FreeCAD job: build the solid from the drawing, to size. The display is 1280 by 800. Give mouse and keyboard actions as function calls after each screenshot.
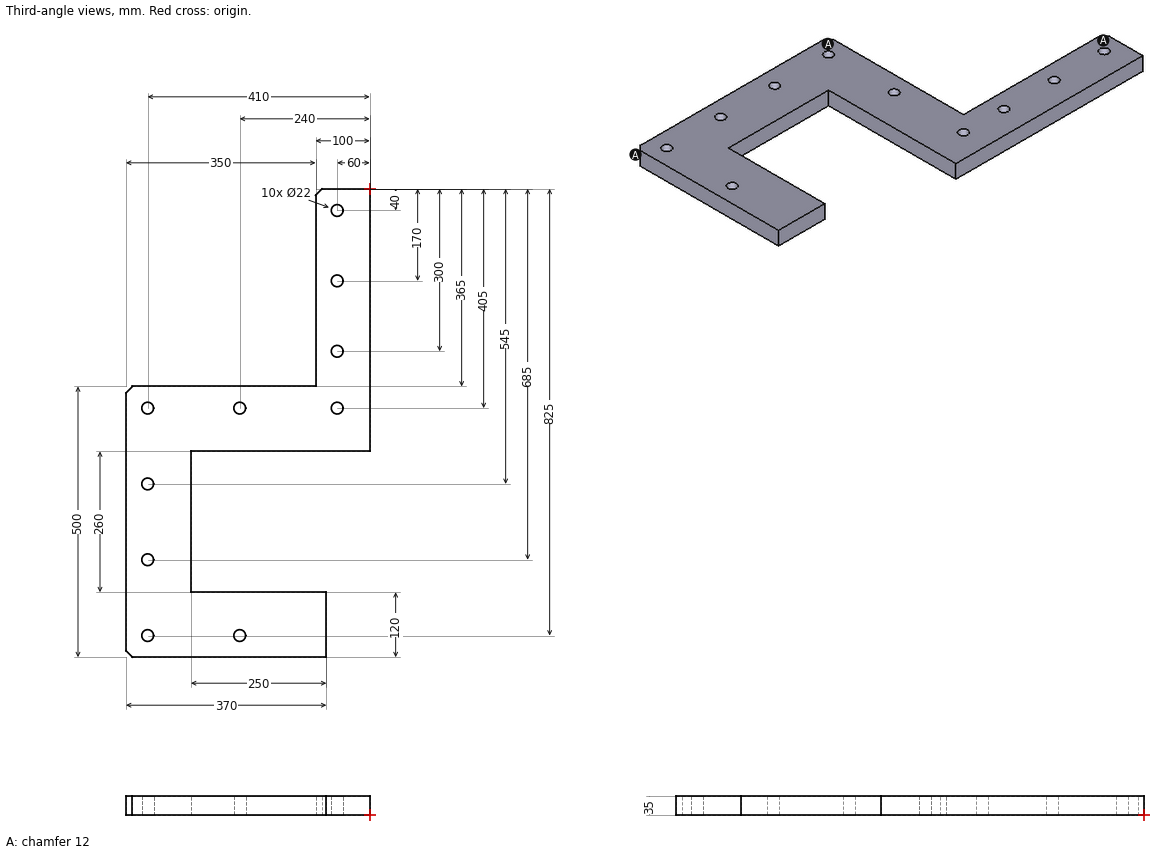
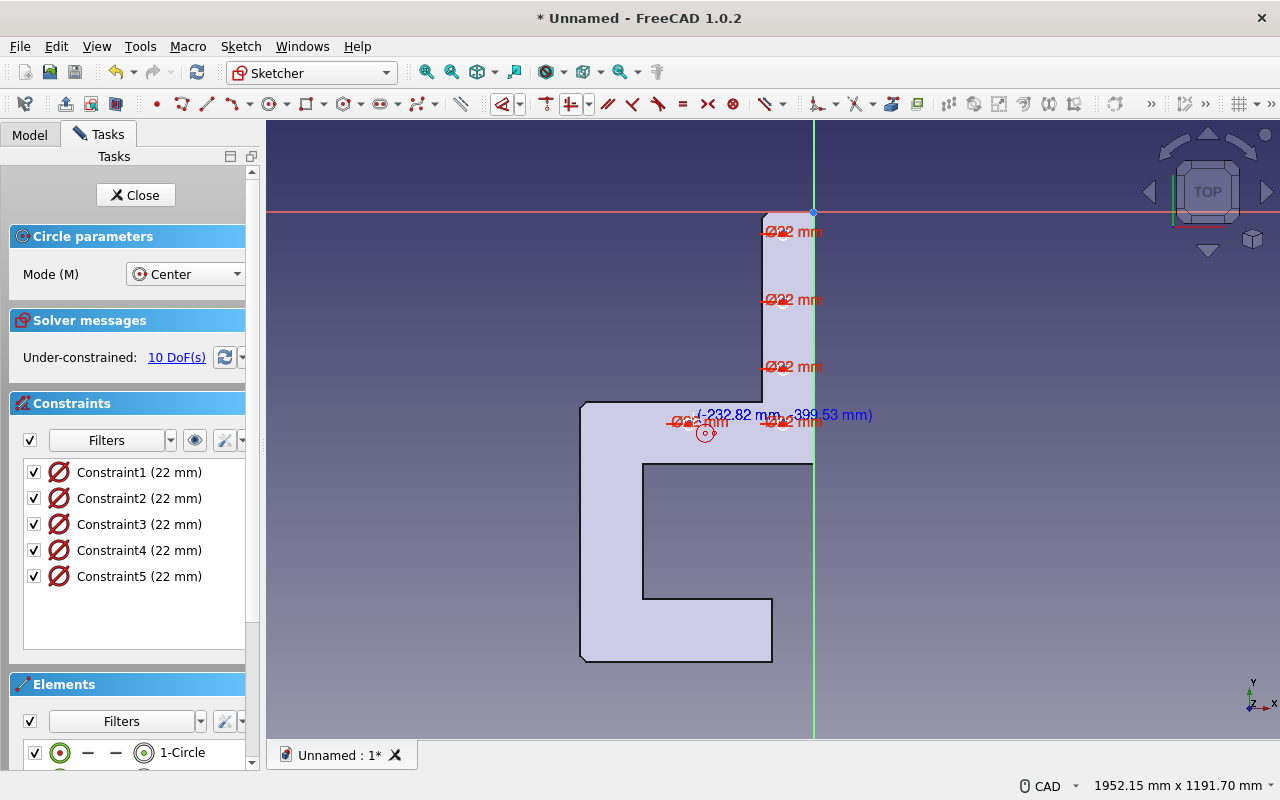
scroll(601, 423, up, 7)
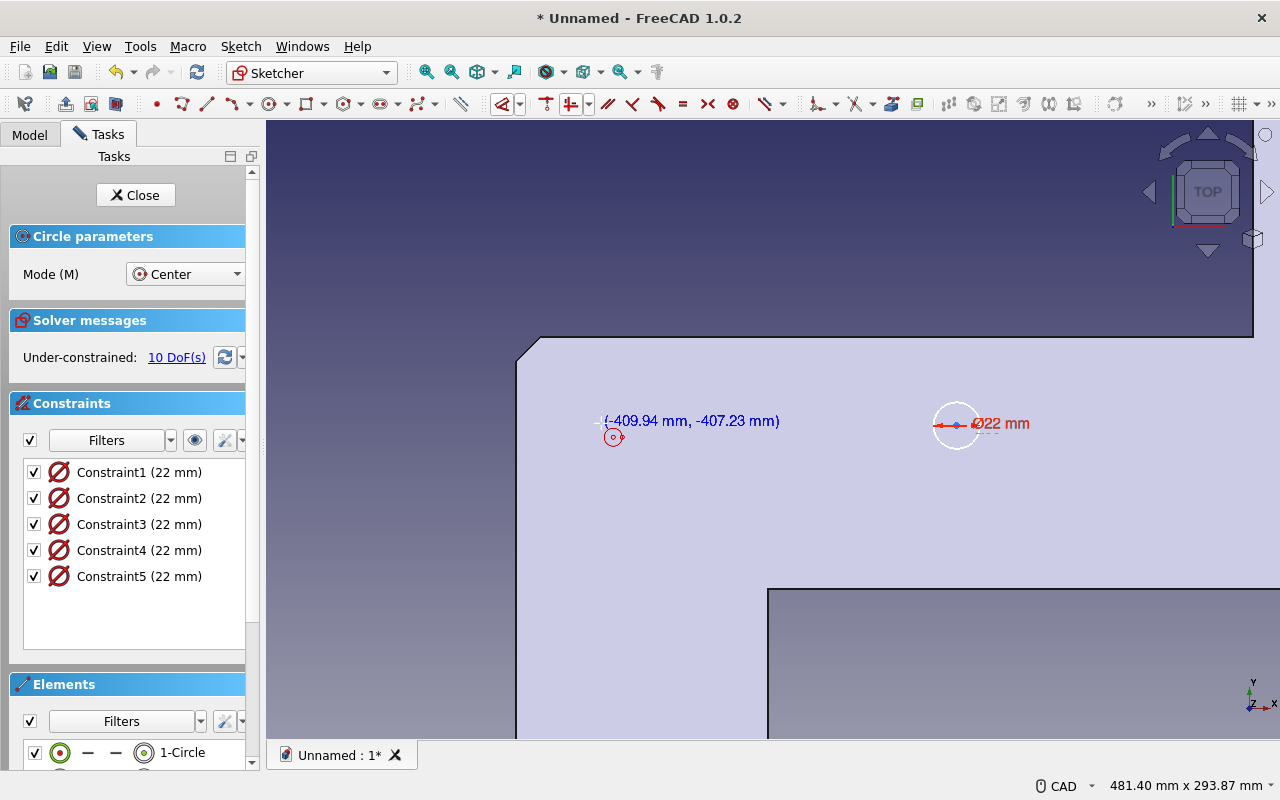
scroll(601, 423, down, 7)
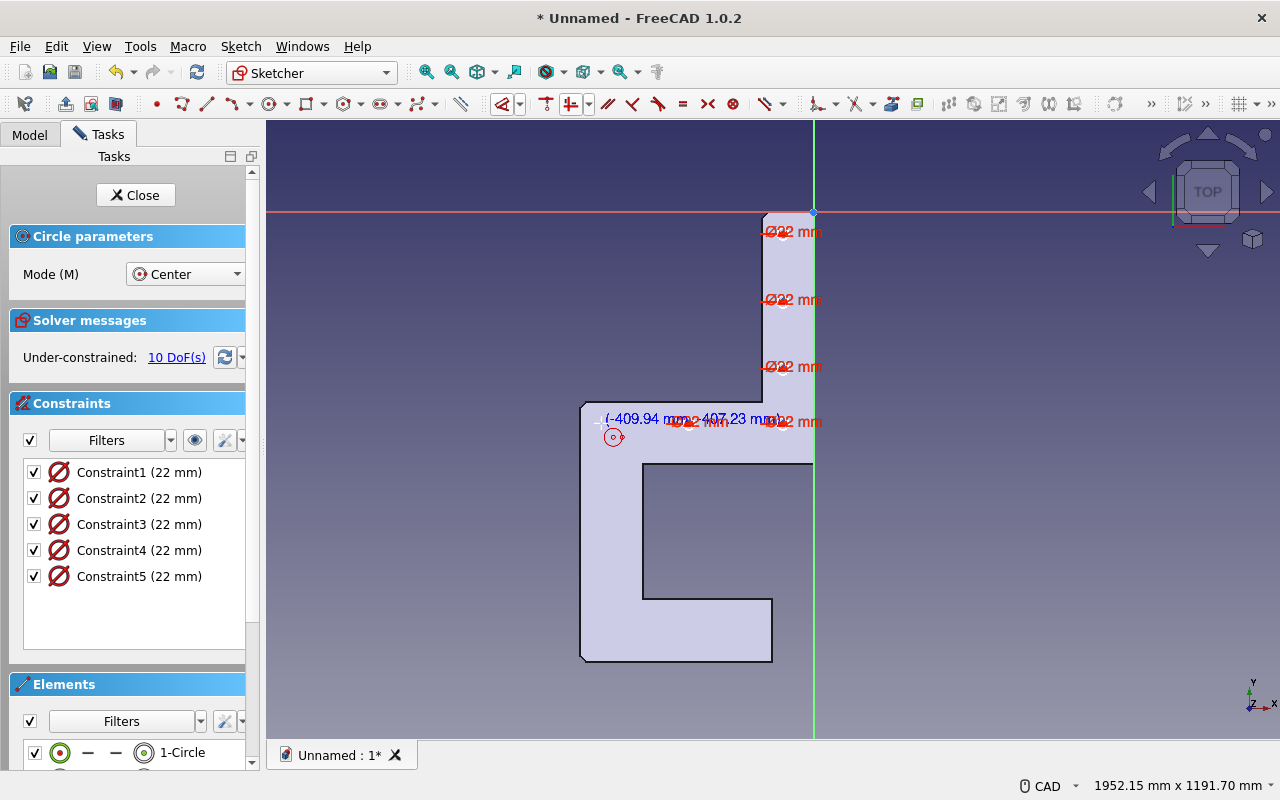
click(601, 423)
move(605, 419)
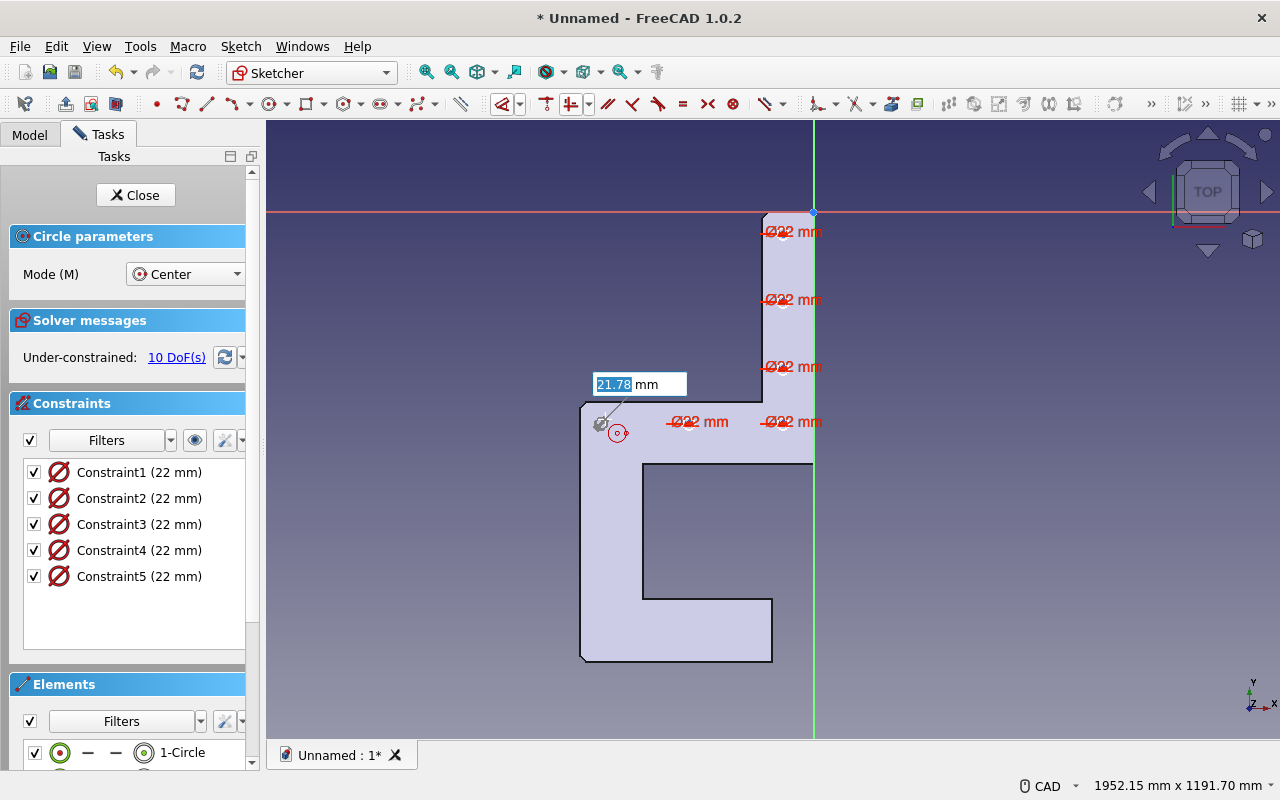
text(22)
key(Return)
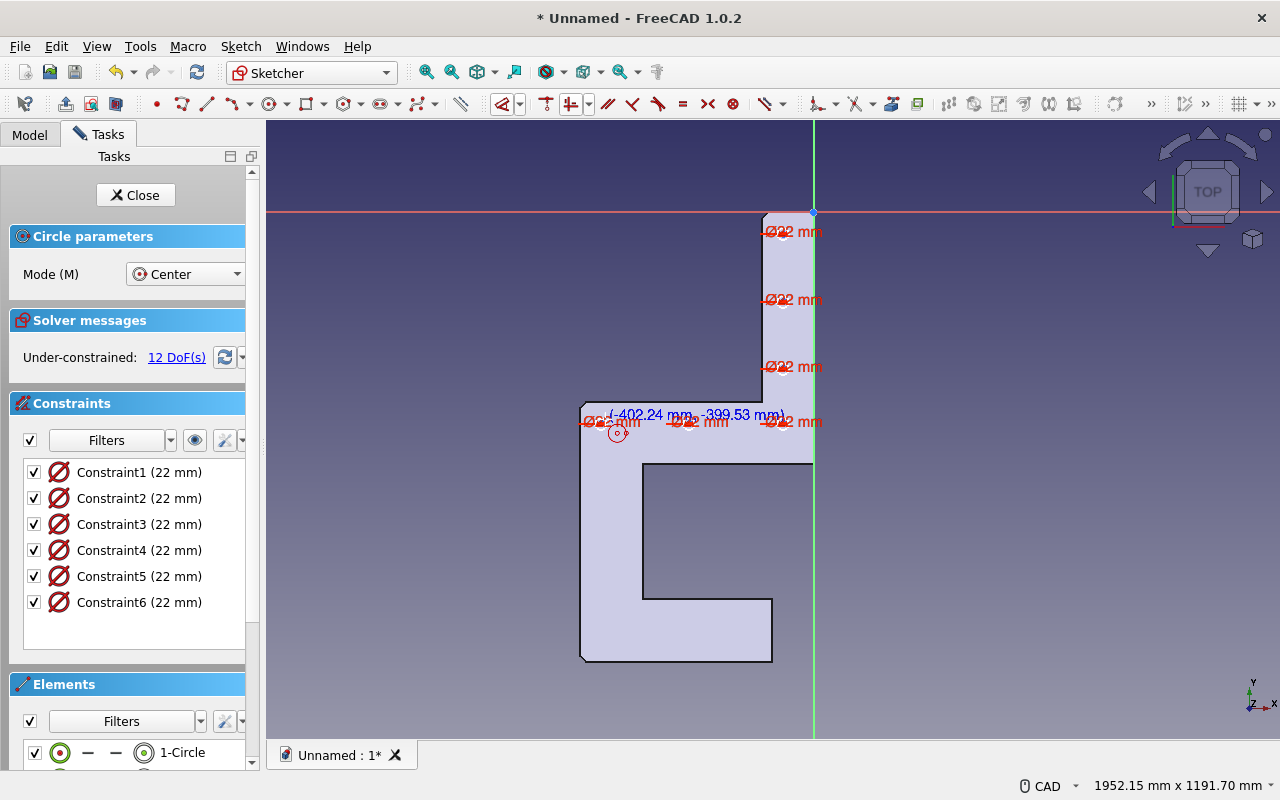
scroll(601, 496, up, 7)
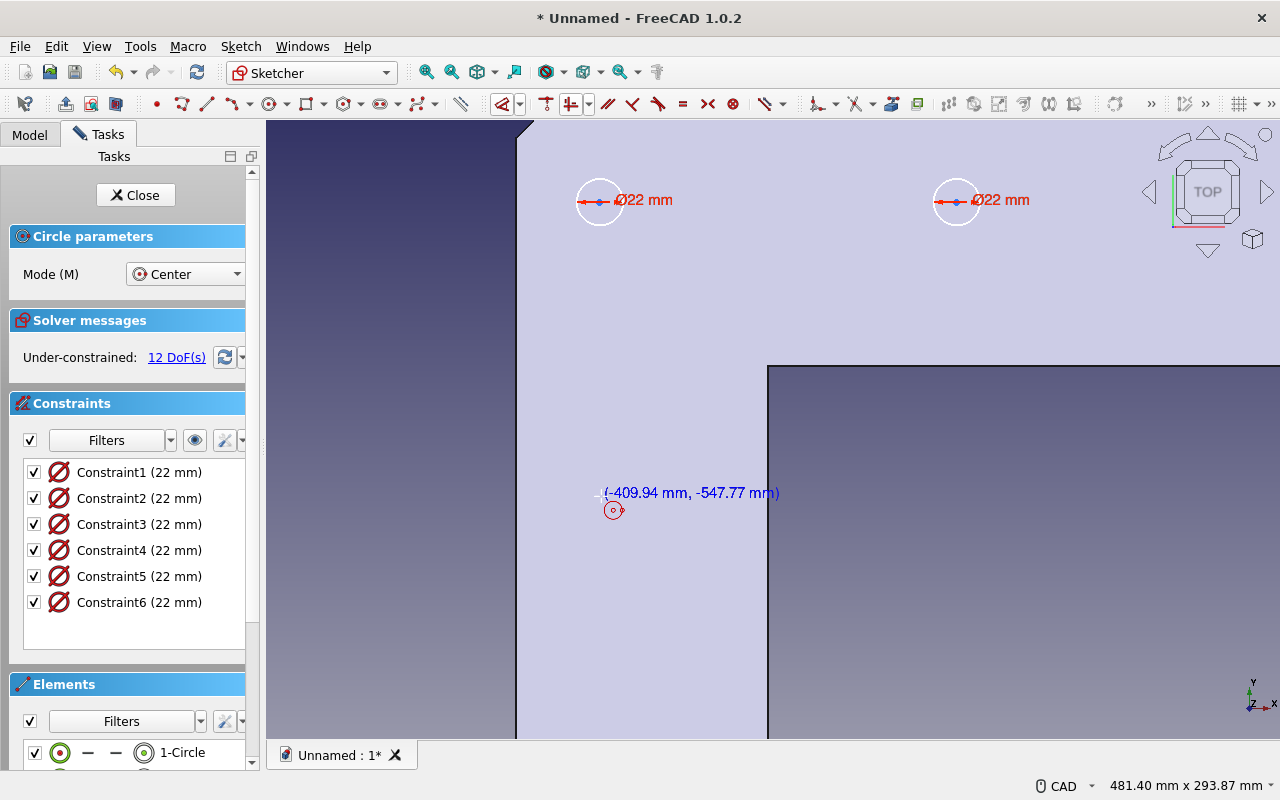
scroll(601, 496, down, 7)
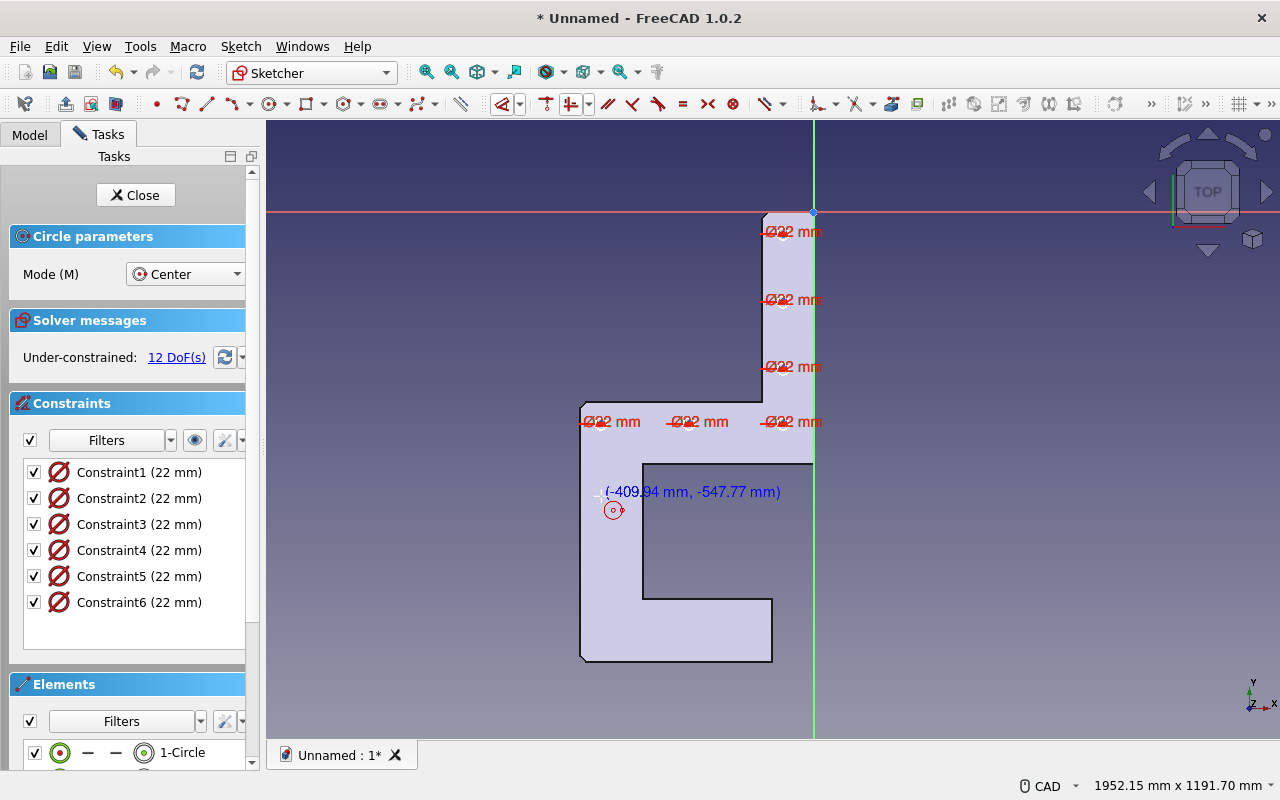
click(601, 496)
move(605, 492)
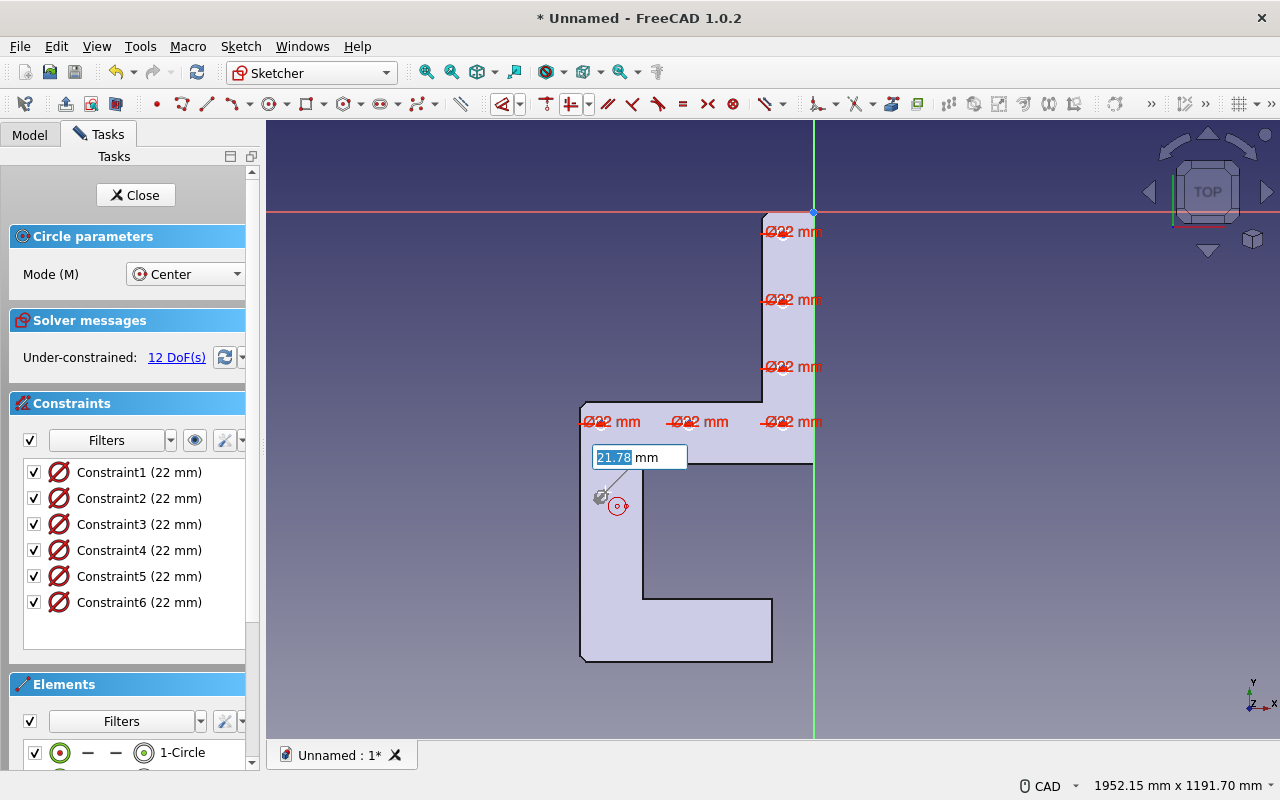
text(22)
key(Return)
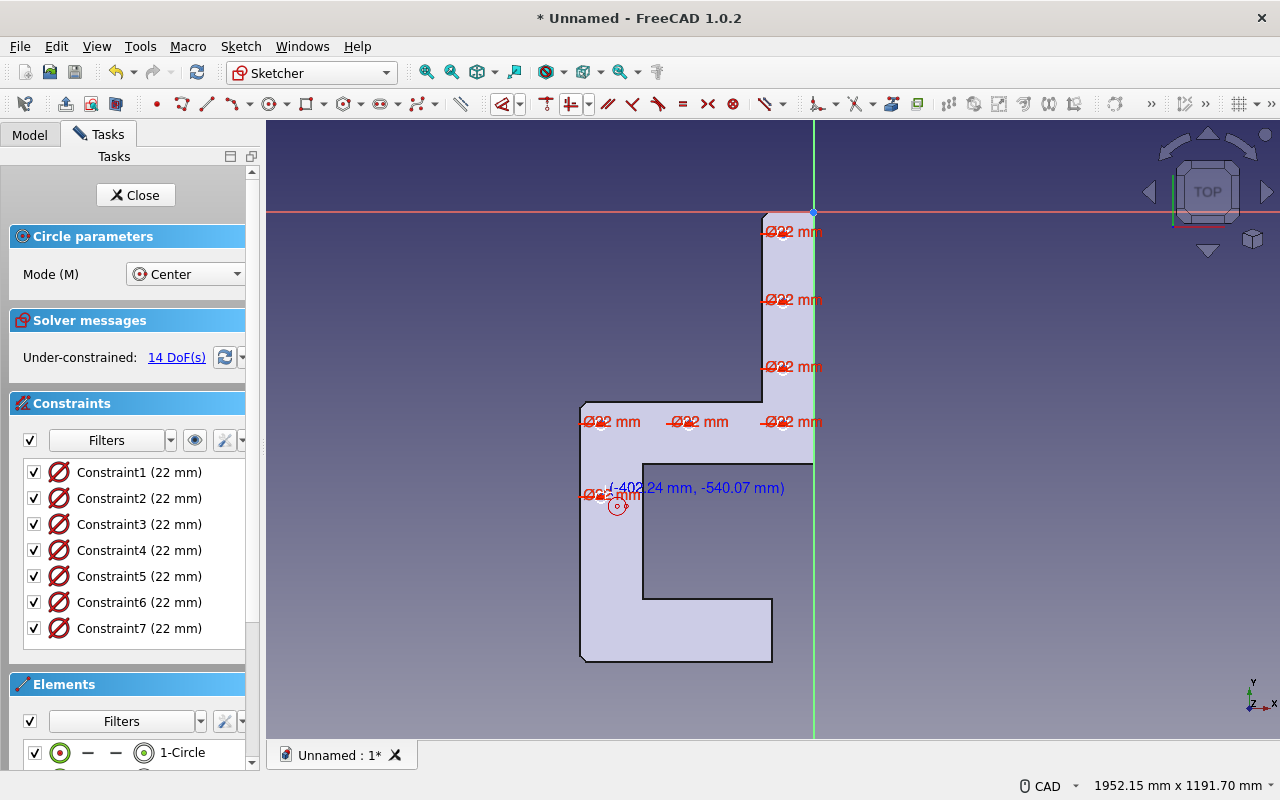
scroll(601, 568, up, 7)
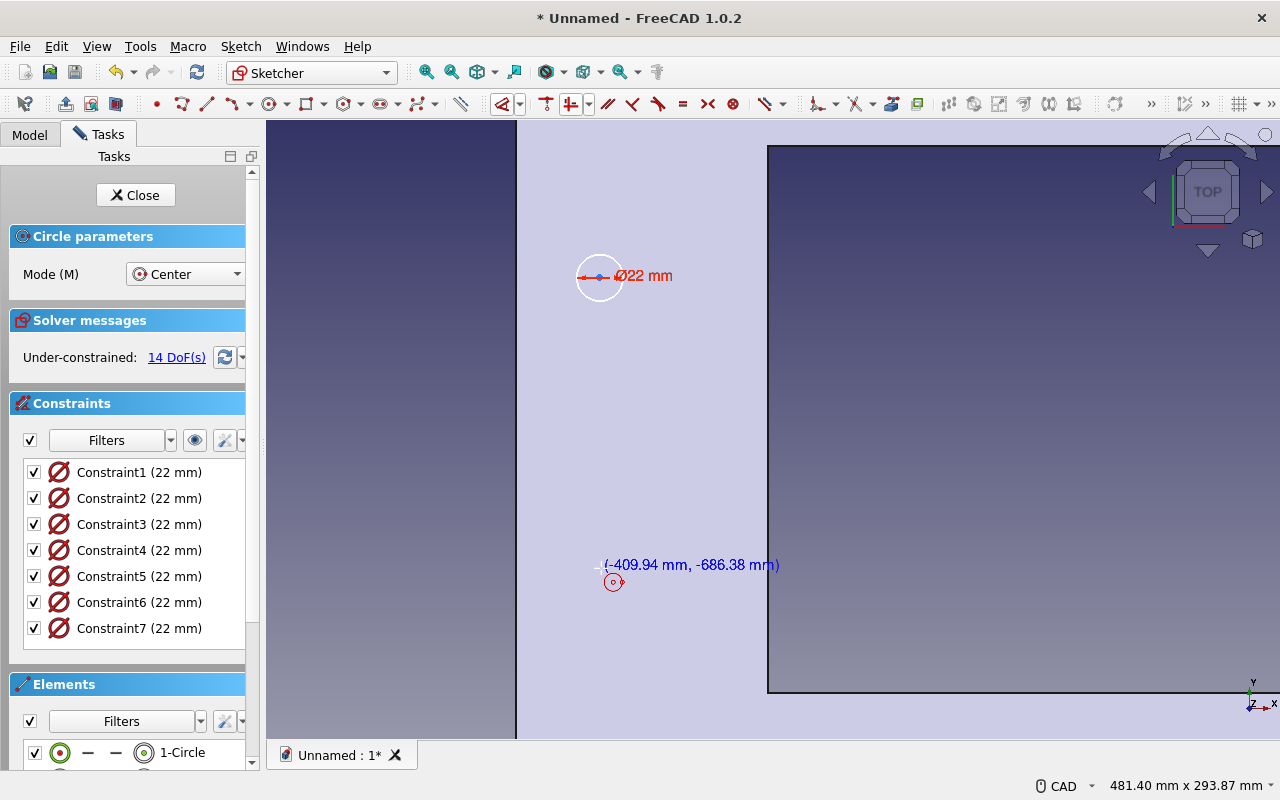
scroll(601, 569, down, 7)